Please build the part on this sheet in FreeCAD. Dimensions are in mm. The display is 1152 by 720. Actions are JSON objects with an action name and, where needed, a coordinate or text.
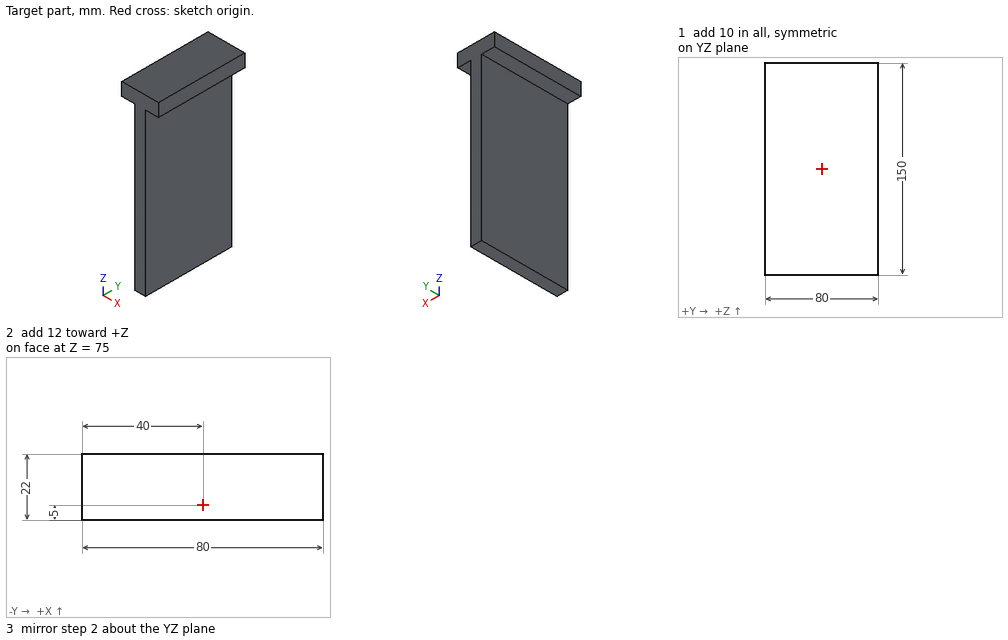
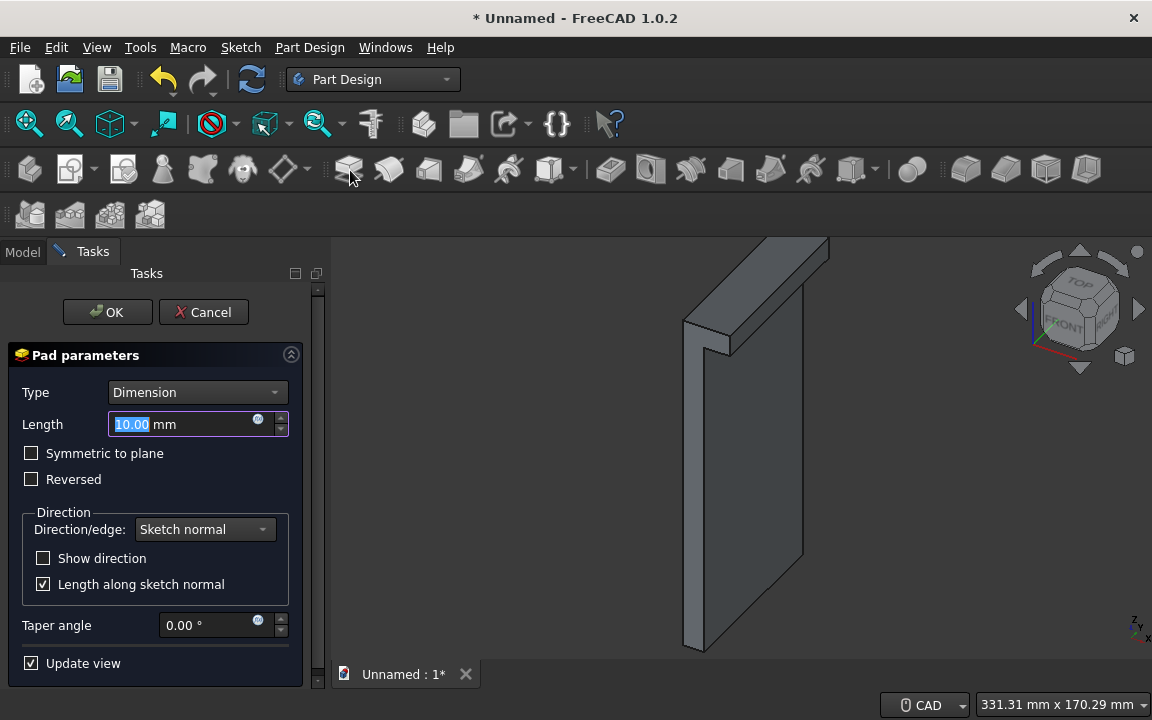
{"action": "type", "text": "12"}
{"action": "key", "text": "Tab"}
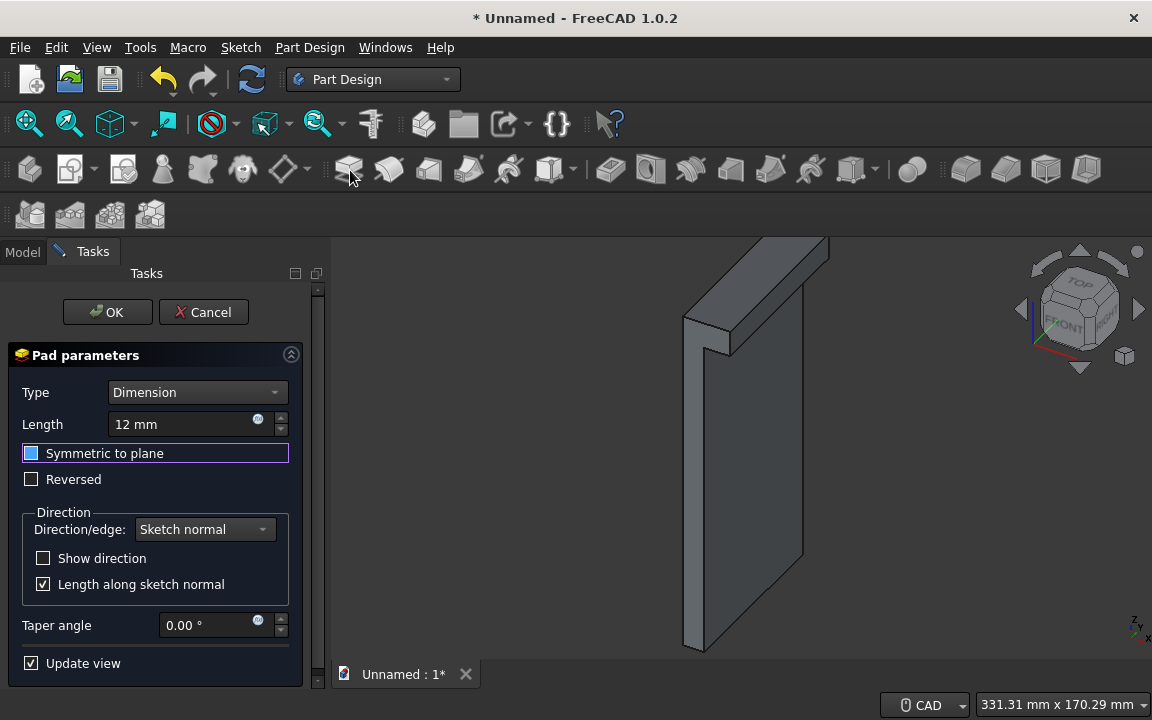
{"action": "left_click", "coordinate": [108, 312]}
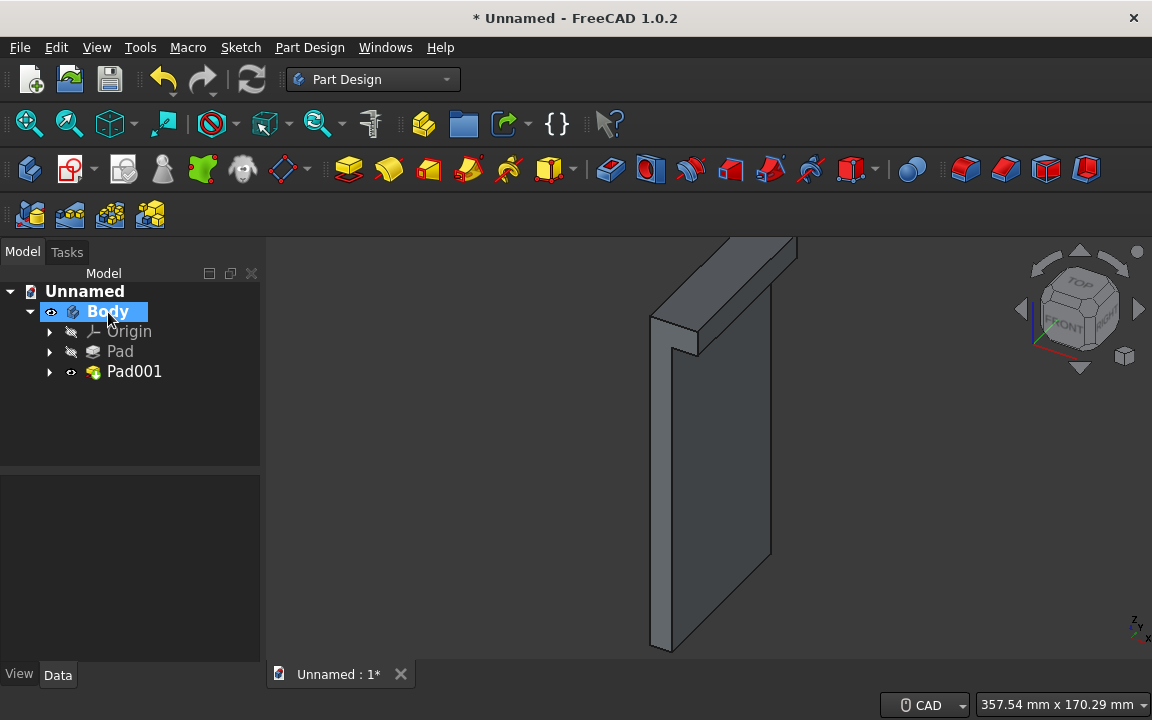
{"action": "left_click", "coordinate": [30, 124]}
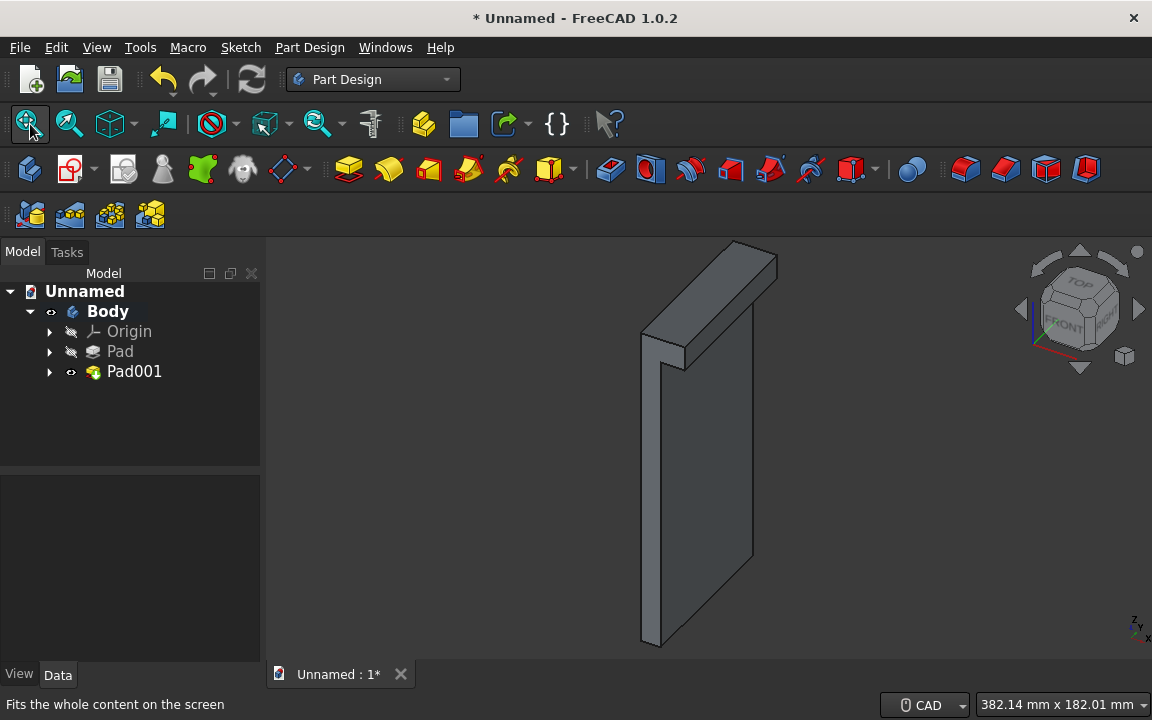
{"action": "left_click", "coordinate": [116, 372]}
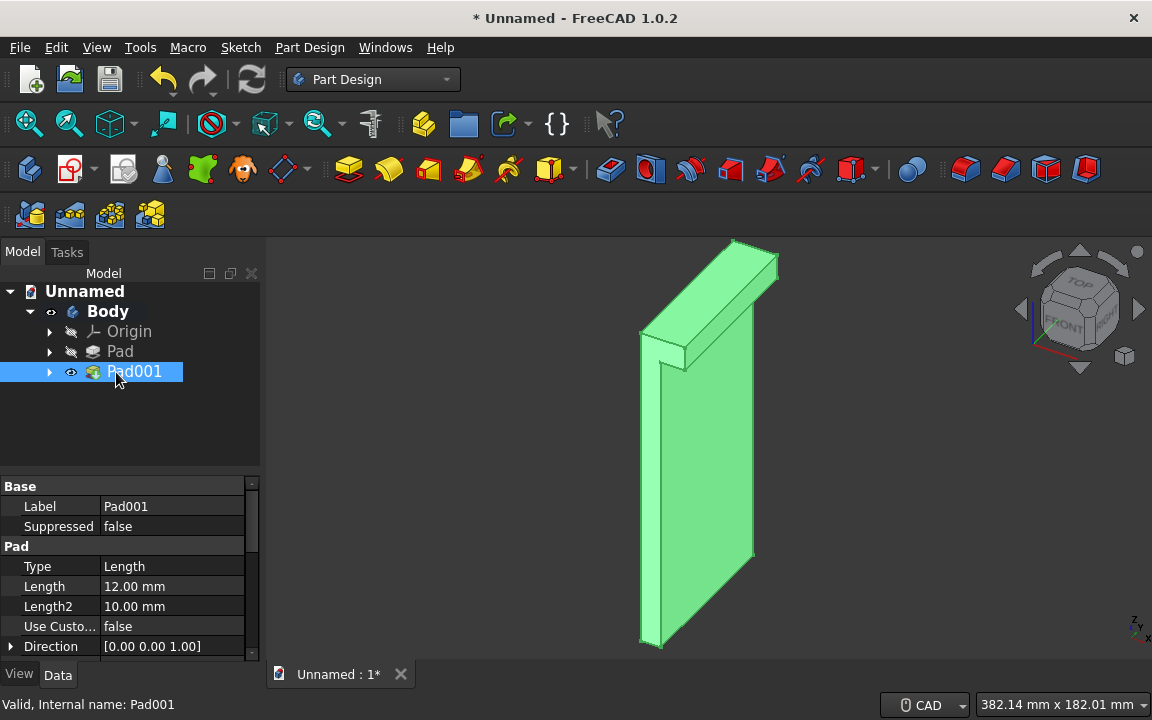
{"action": "left_click", "coordinate": [30, 214]}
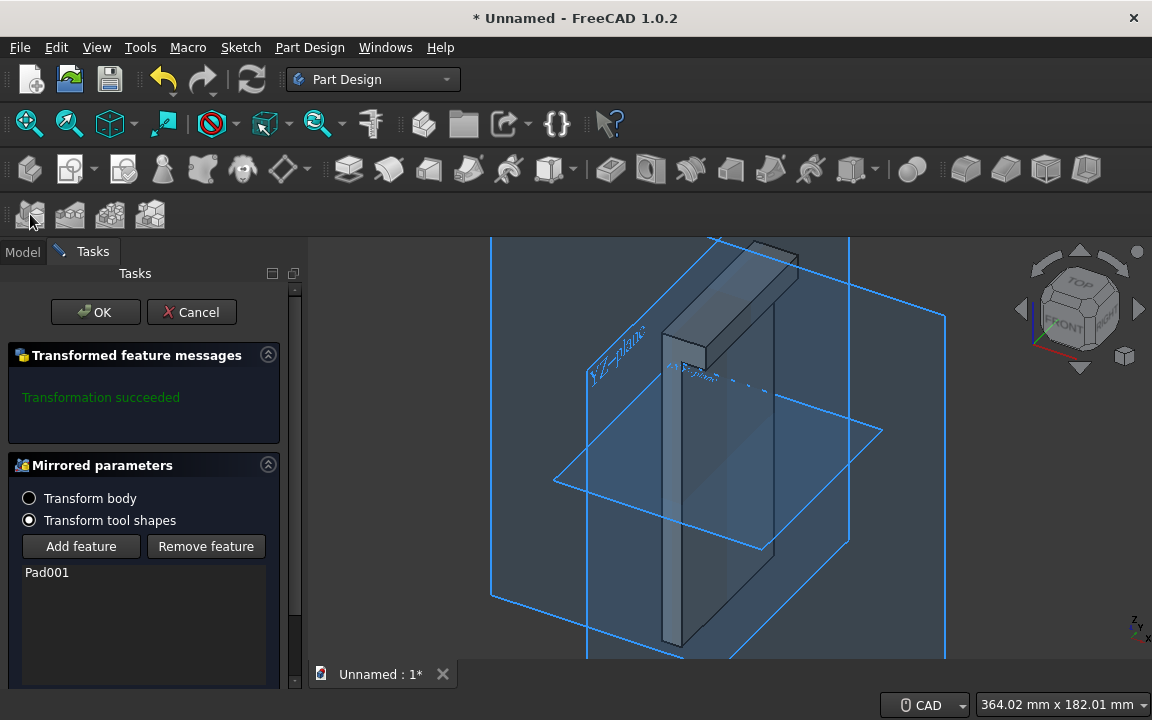
{"action": "scroll", "coordinate": [295, 486], "scroll_direction": "down", "scroll_amount": 2}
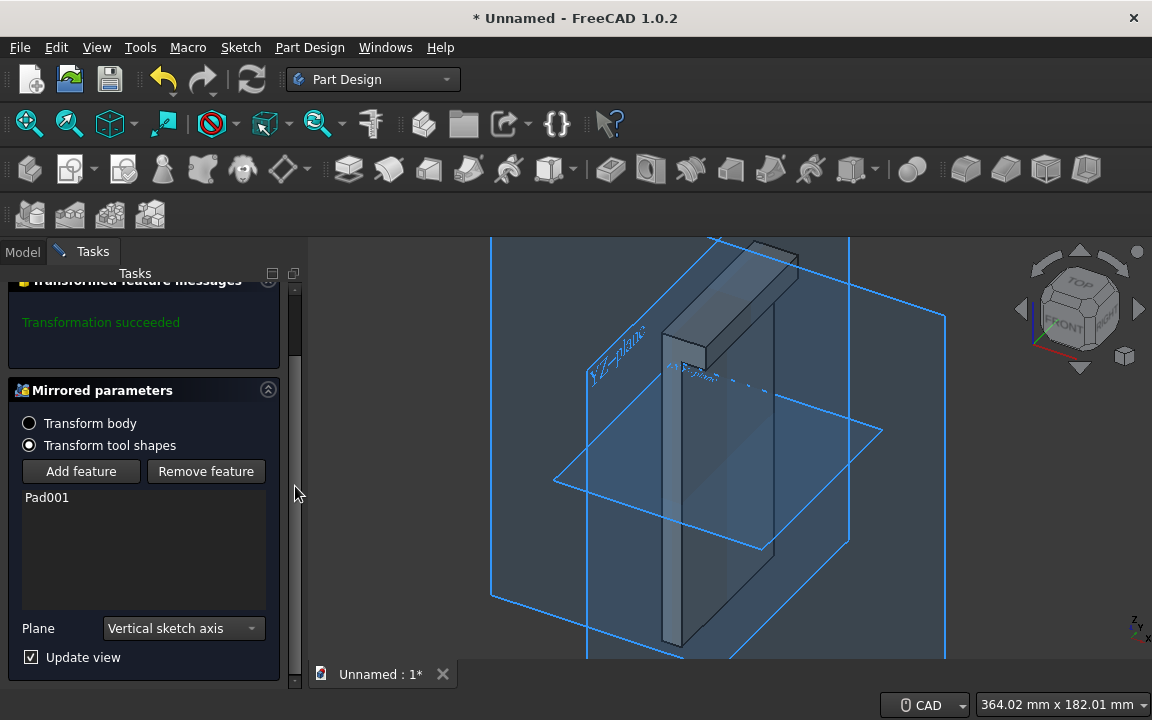
{"action": "left_click", "coordinate": [184, 628]}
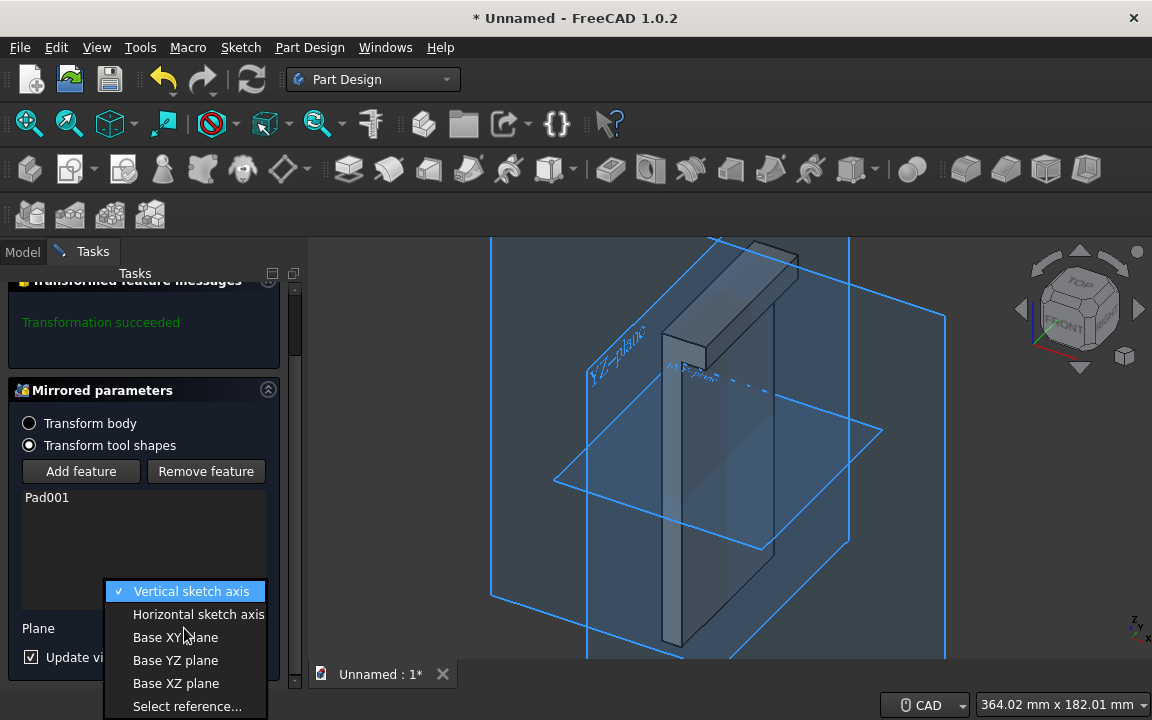
{"action": "left_click", "coordinate": [184, 660]}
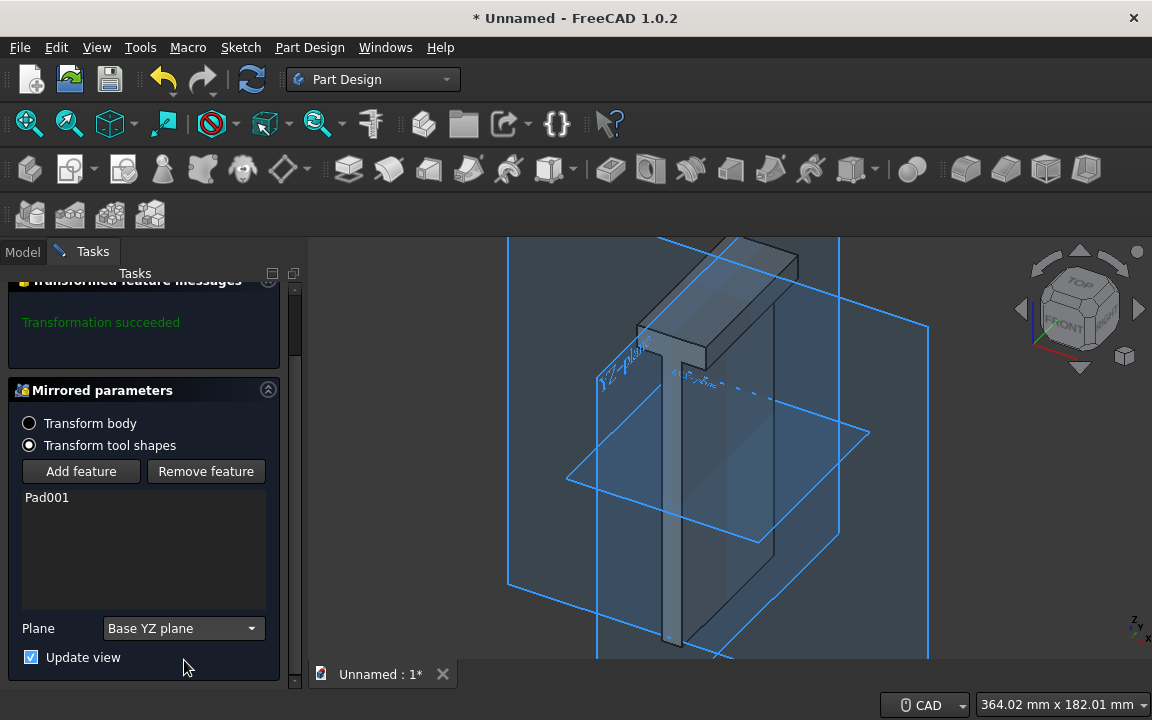
{"action": "scroll", "coordinate": [295, 486], "scroll_direction": "up", "scroll_amount": 2}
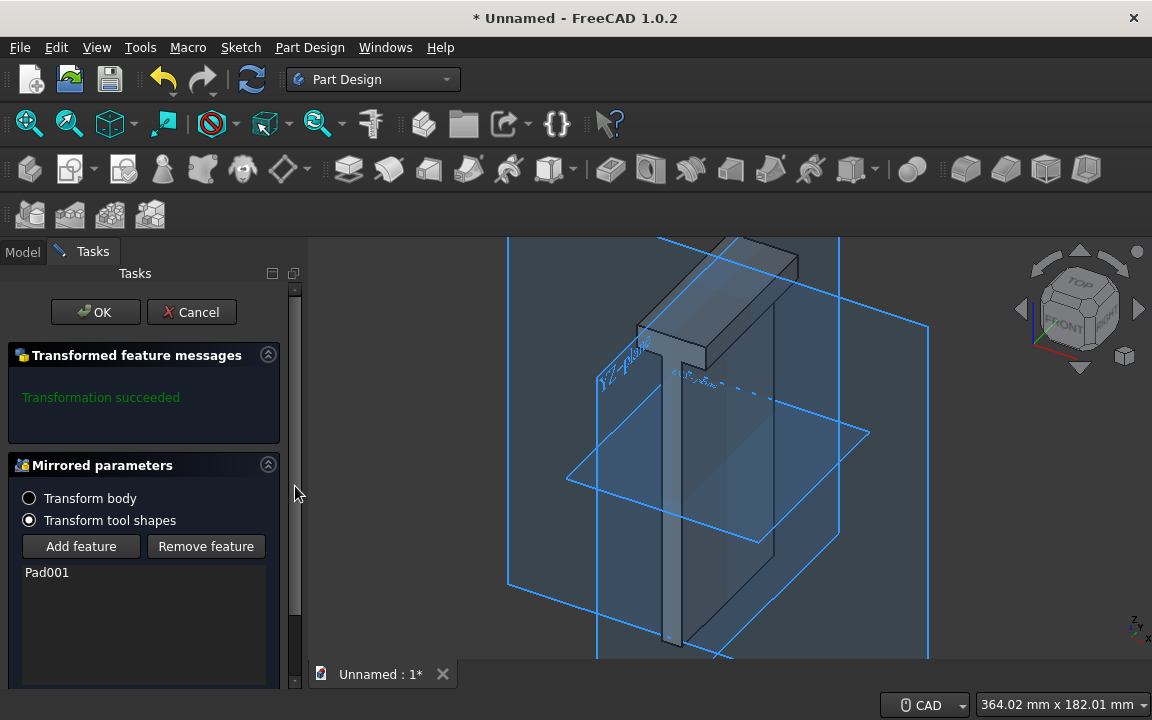
{"action": "left_click", "coordinate": [96, 312]}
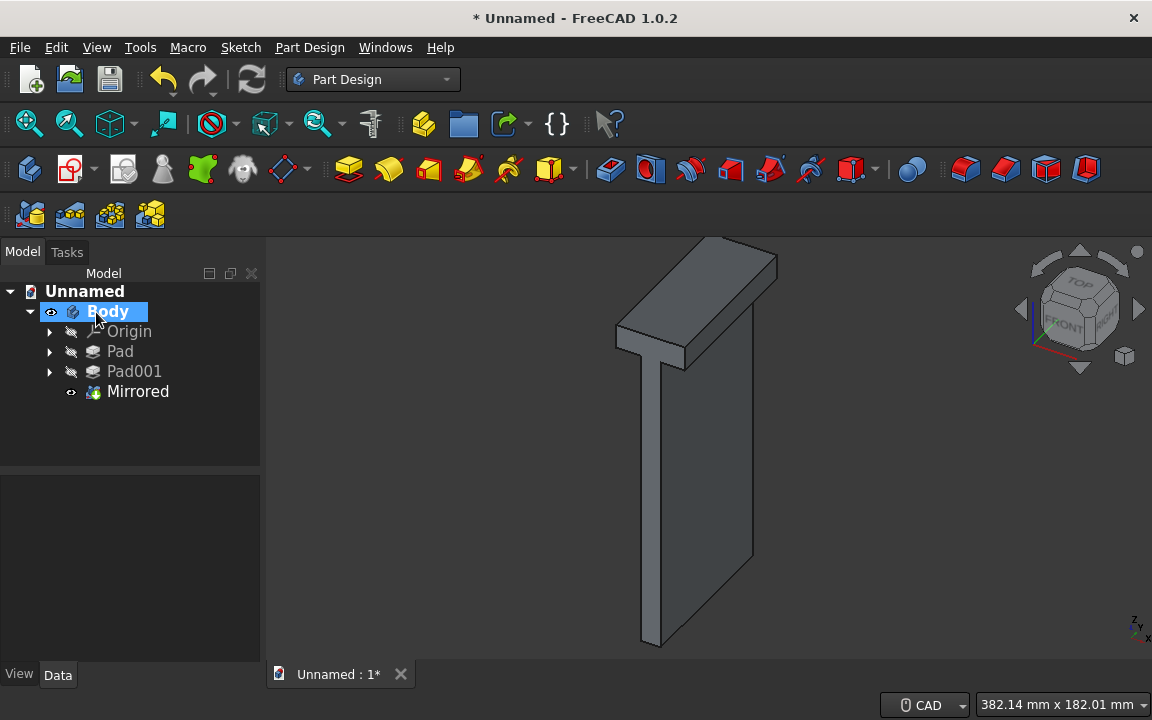
{"action": "key", "text": "0"}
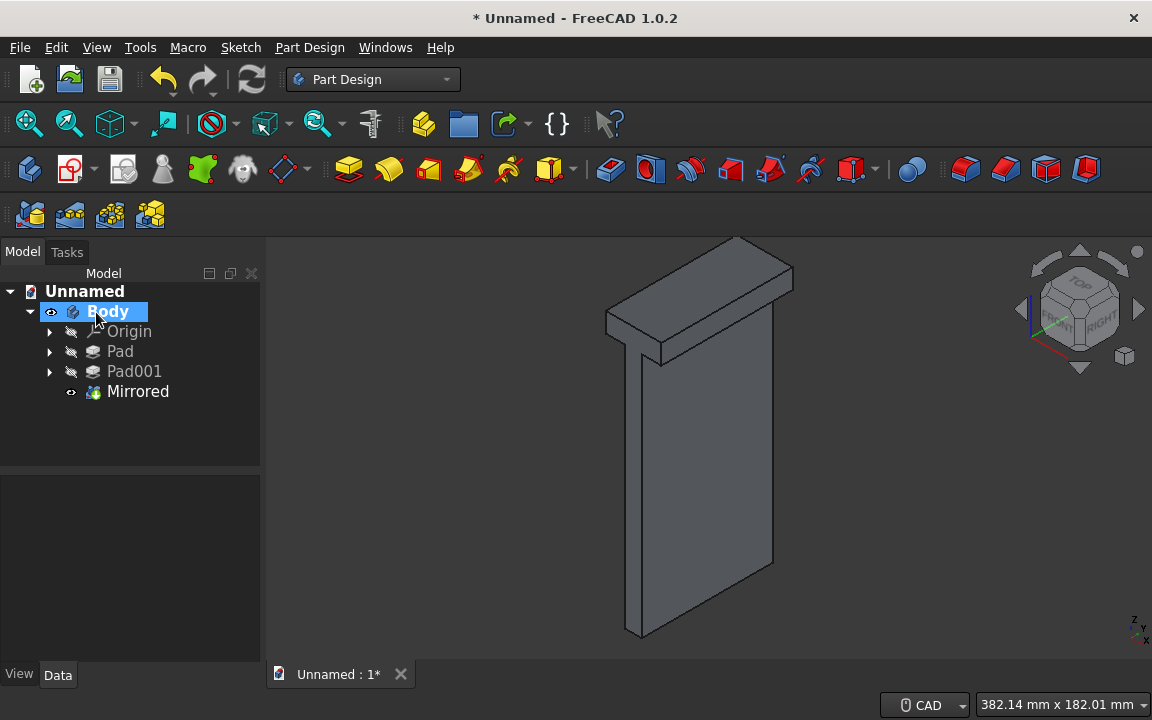
{"action": "left_click", "coordinate": [30, 124]}